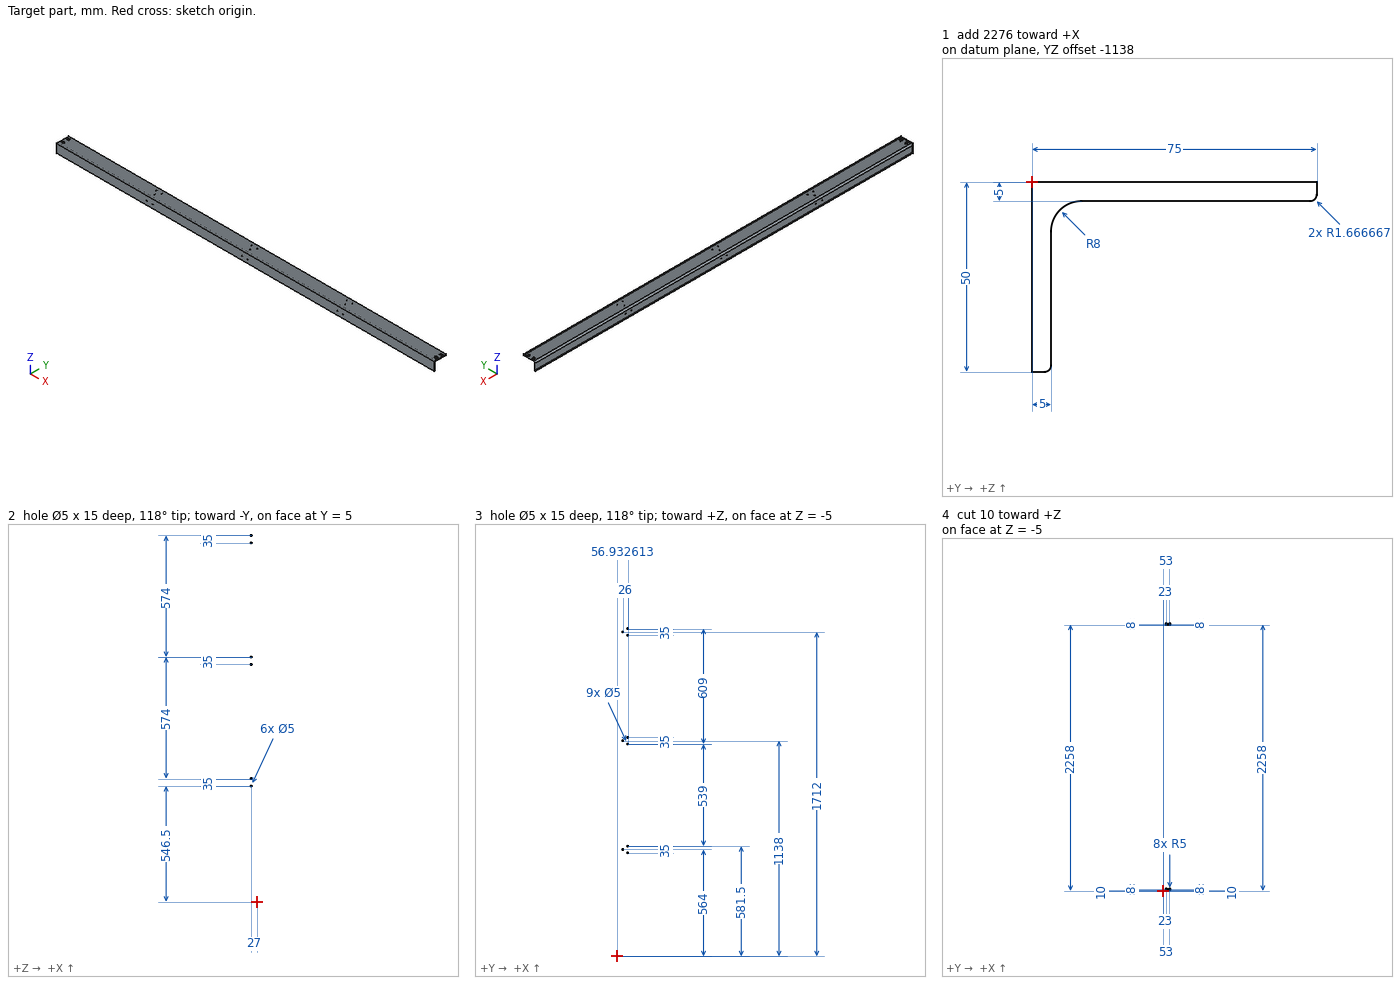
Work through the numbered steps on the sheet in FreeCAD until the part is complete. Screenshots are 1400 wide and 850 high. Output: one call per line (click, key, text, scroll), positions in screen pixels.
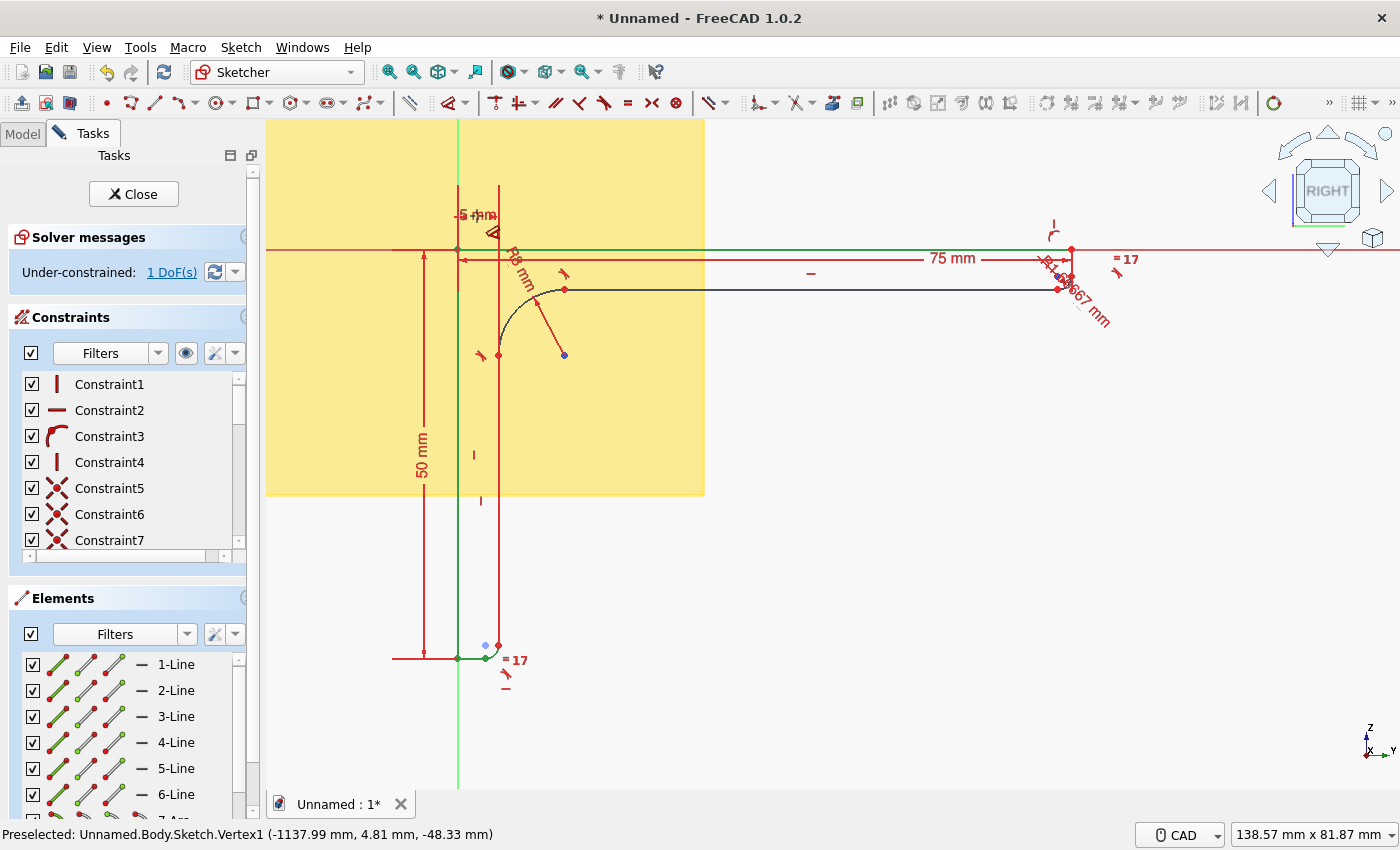
click(564, 290)
click(424, 270)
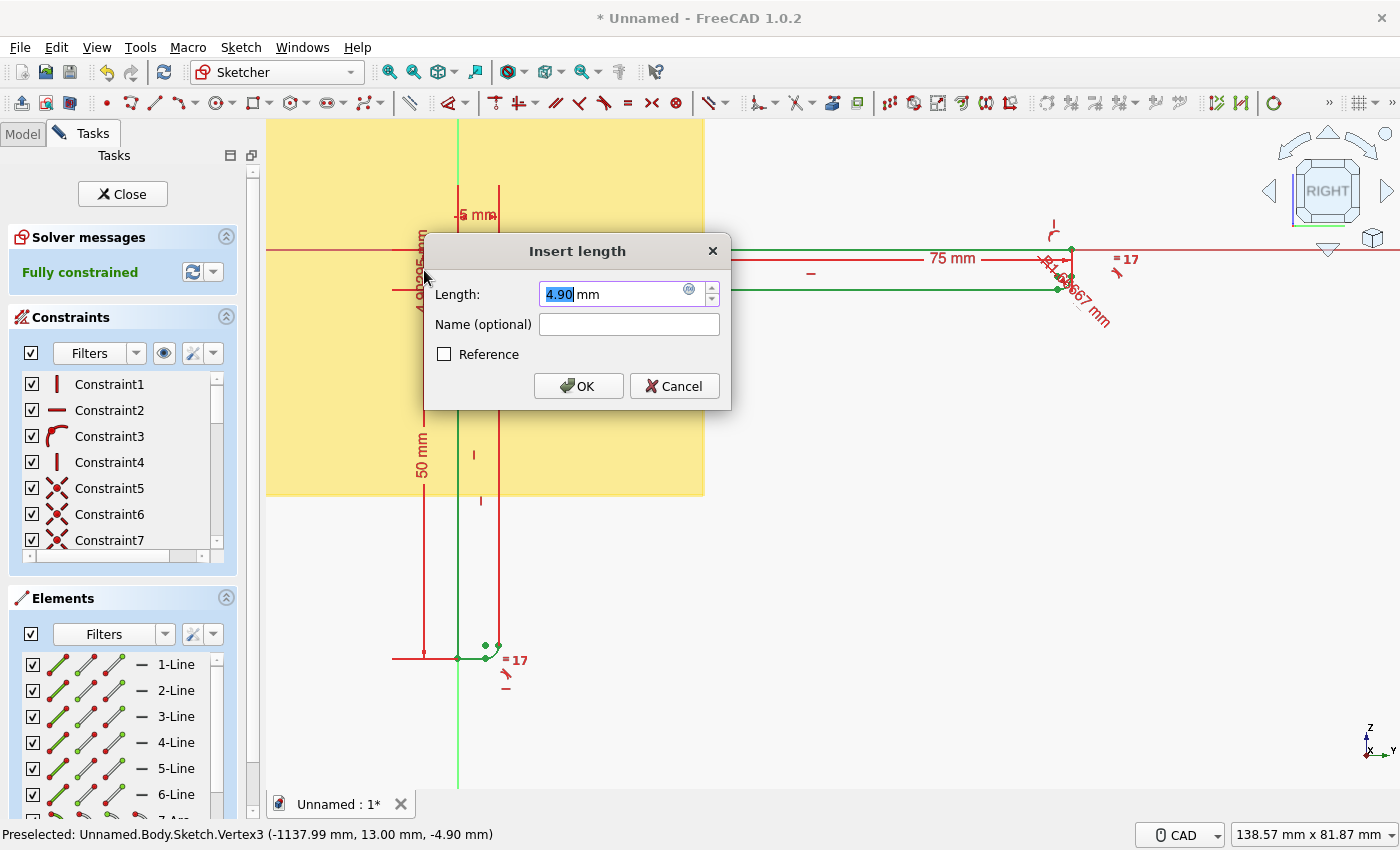
text(5)
key(Return)
key(Escape)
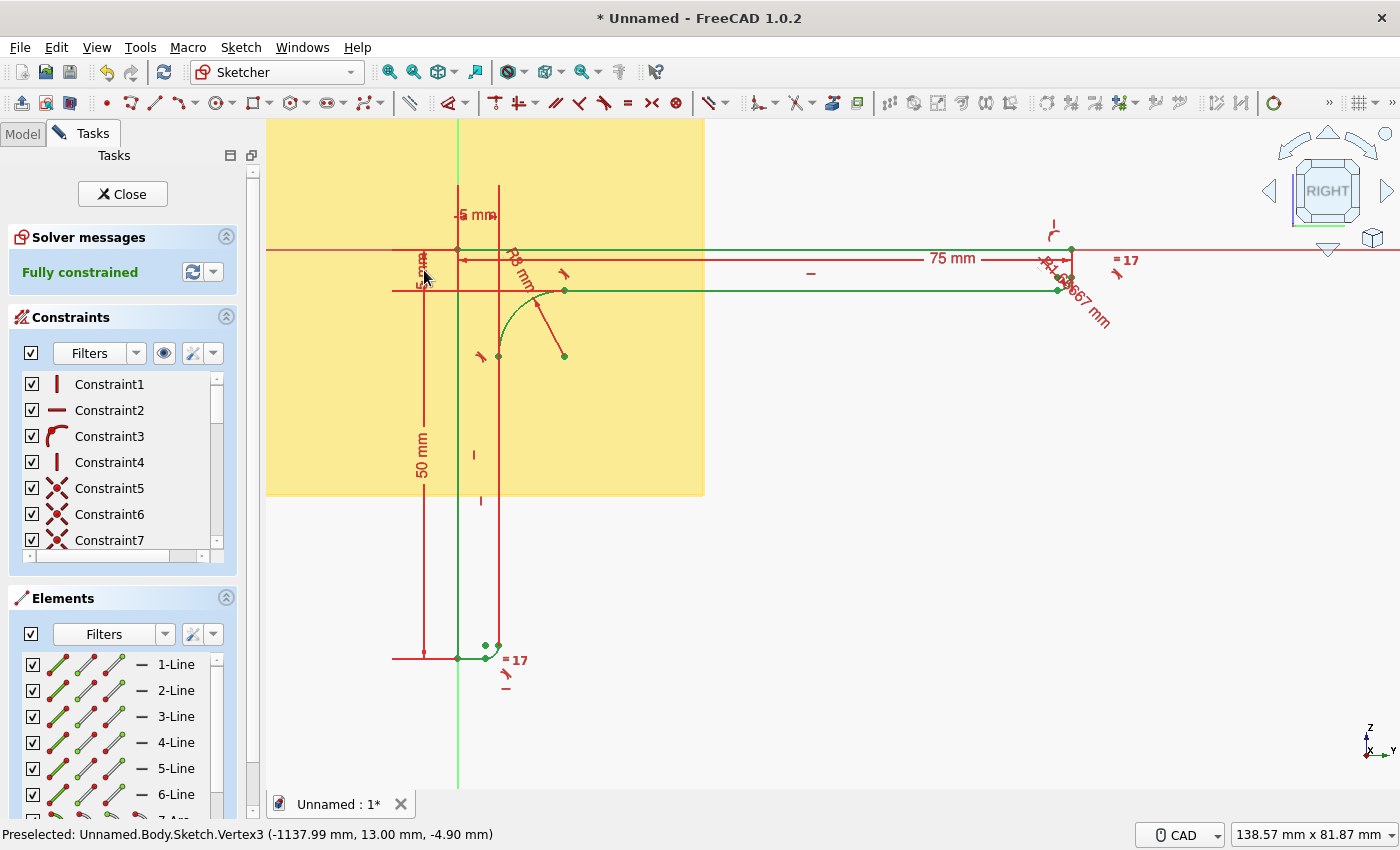
click(123, 194)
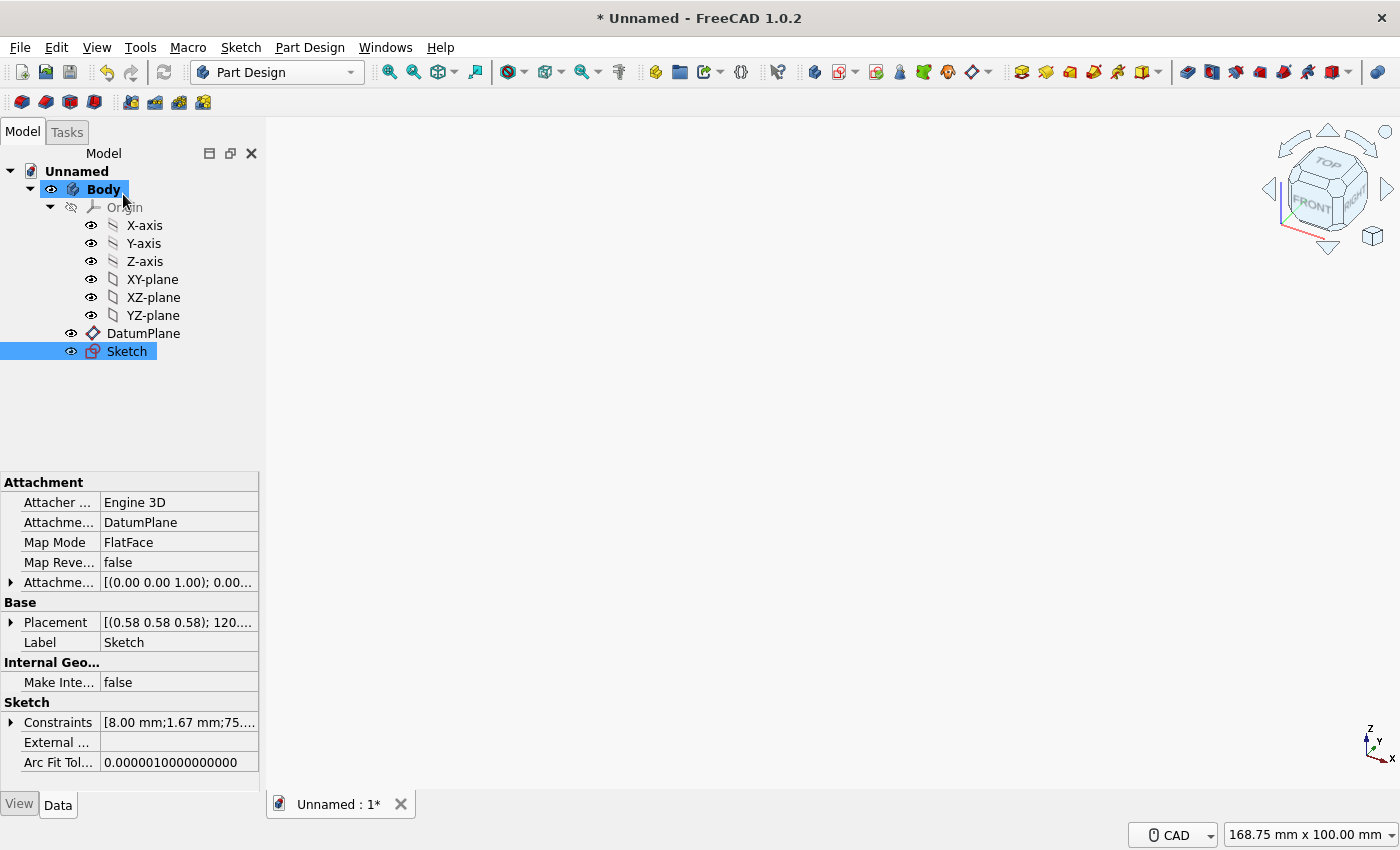
click(1022, 72)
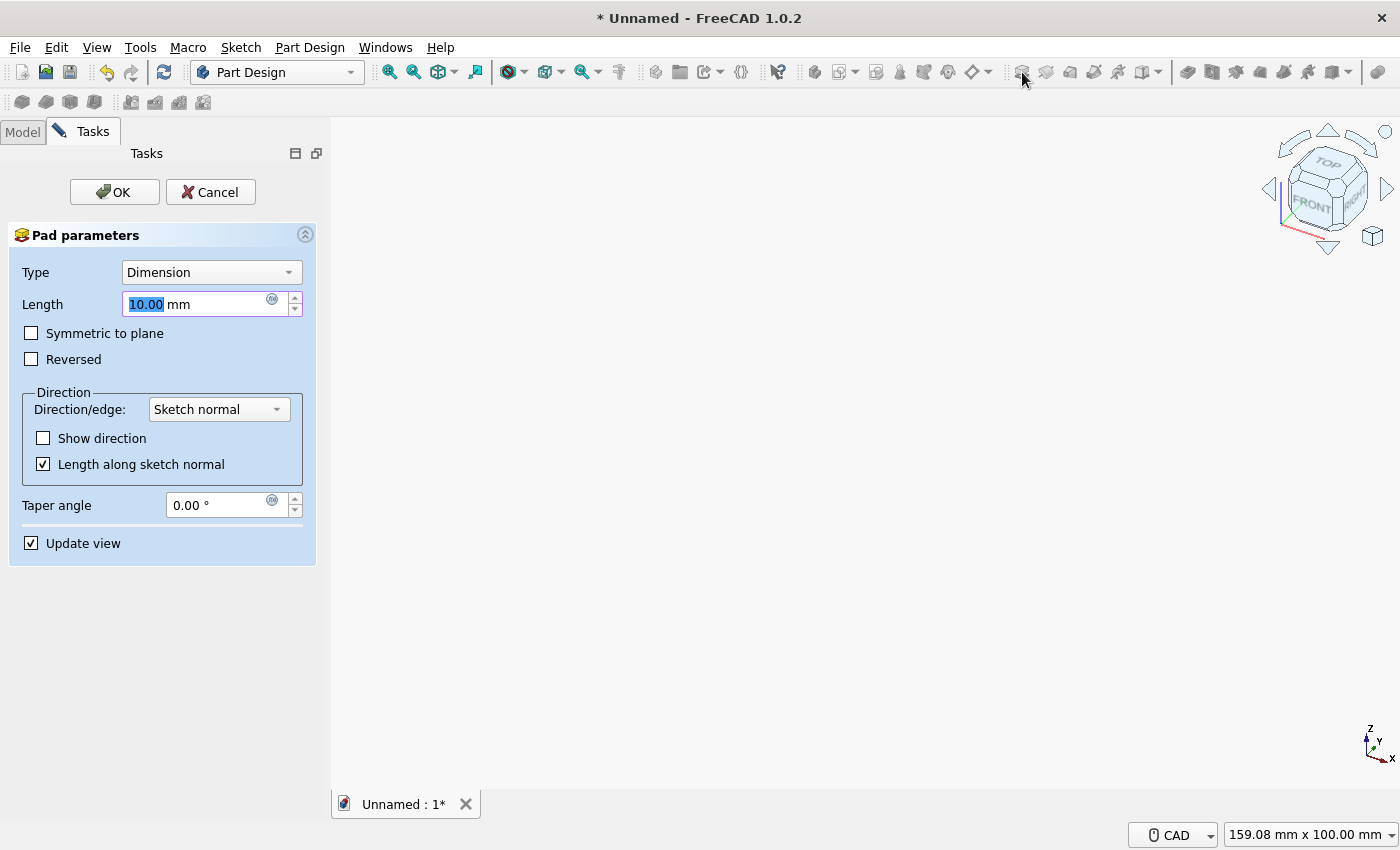
text(2276)
key(Tab)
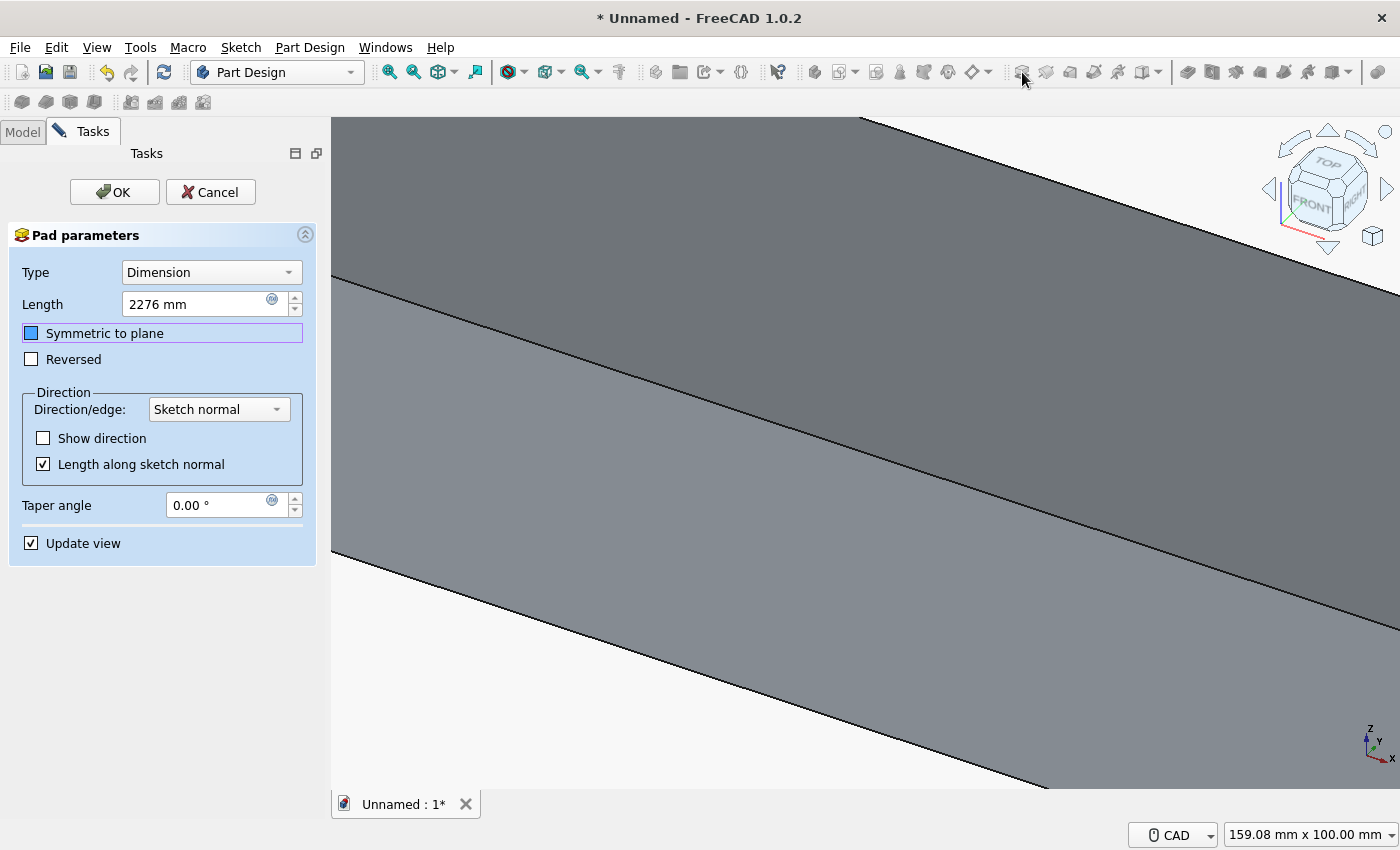
click(115, 192)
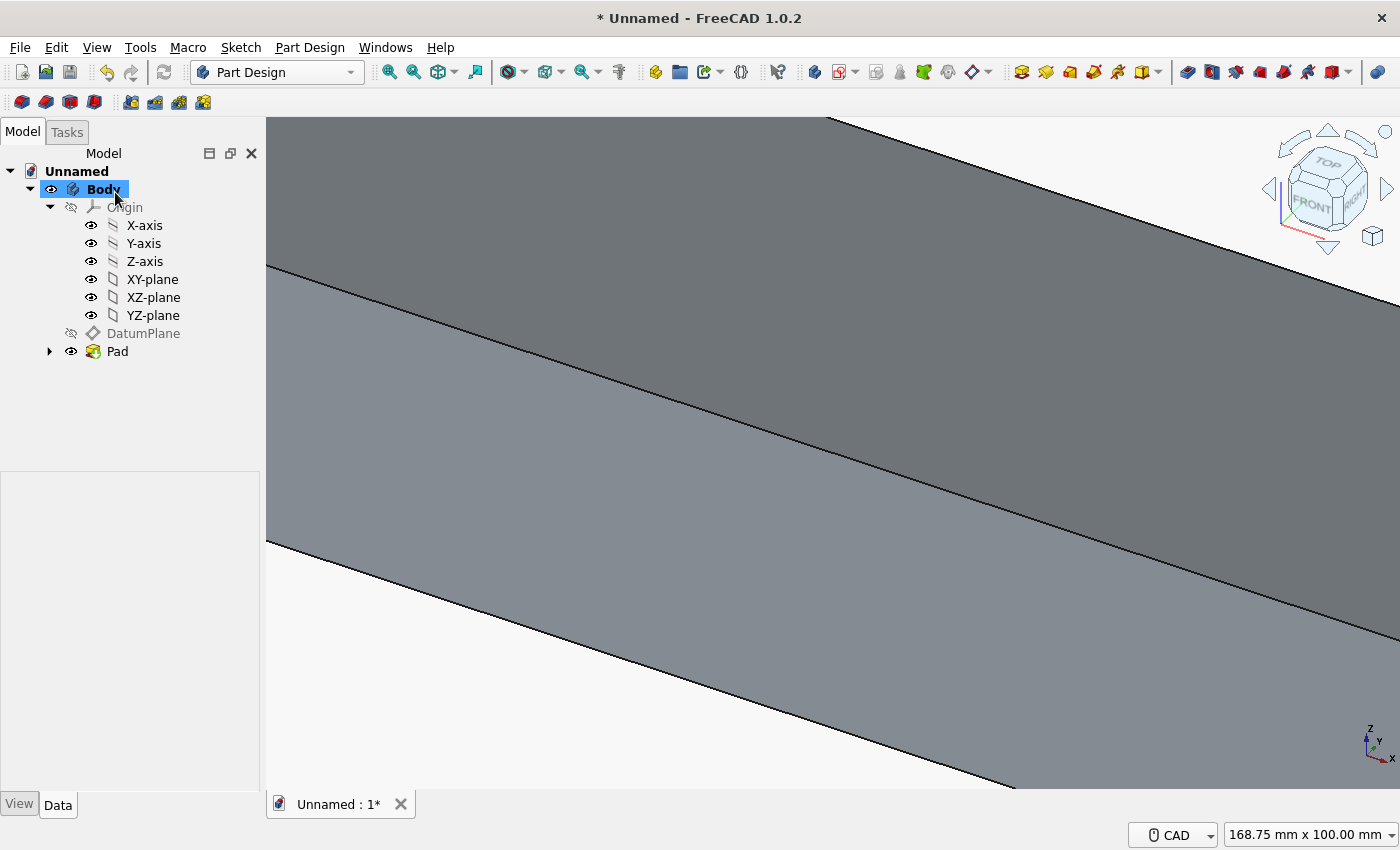
click(390, 72)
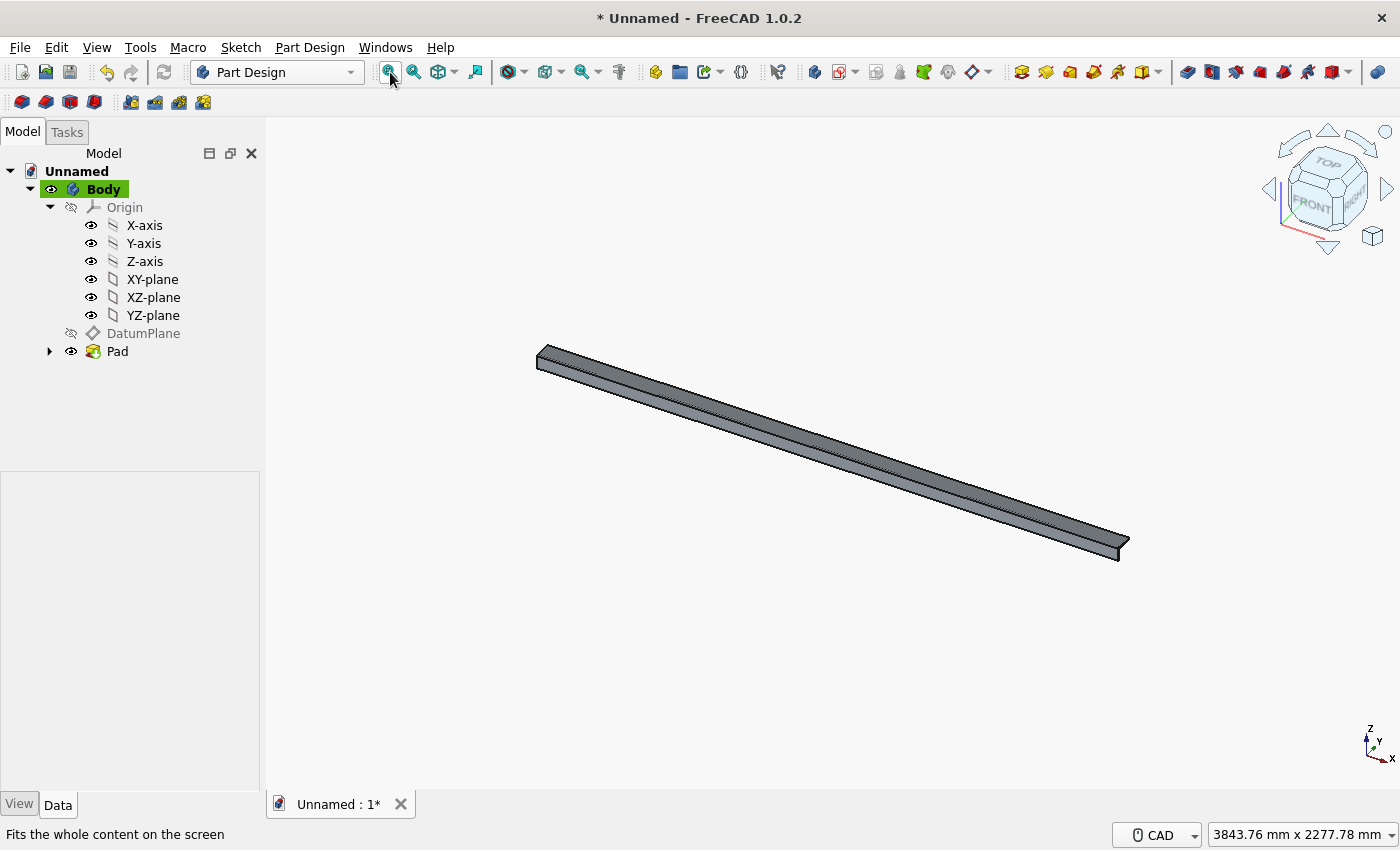
key(4)